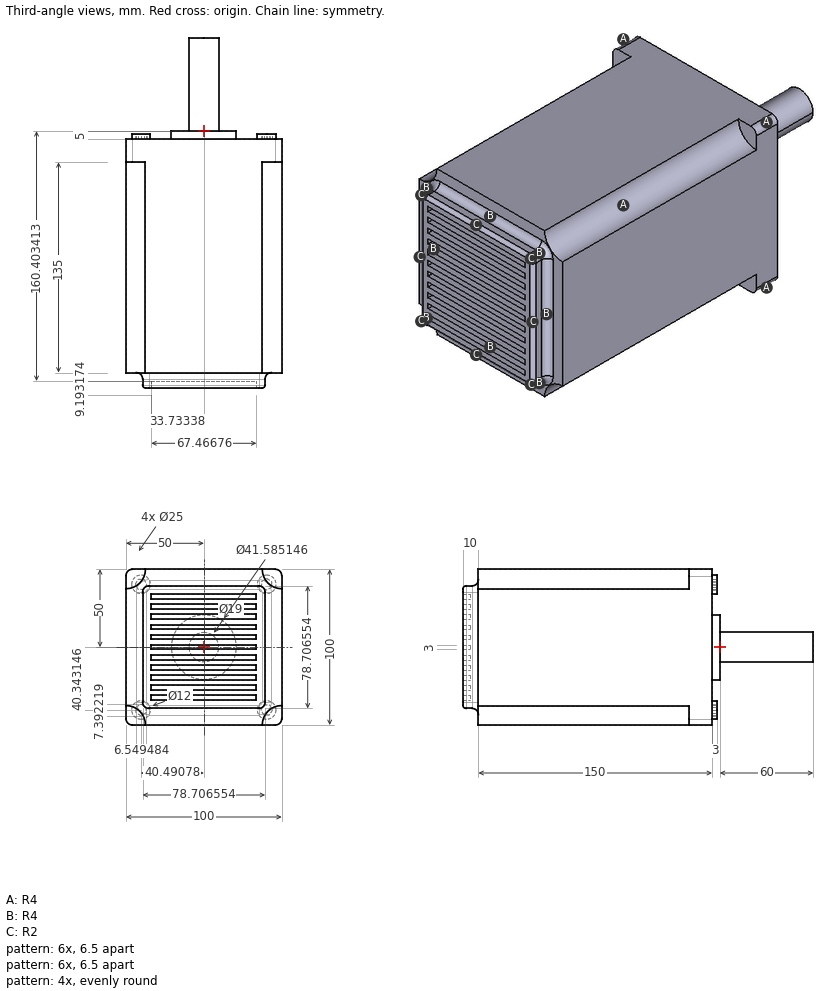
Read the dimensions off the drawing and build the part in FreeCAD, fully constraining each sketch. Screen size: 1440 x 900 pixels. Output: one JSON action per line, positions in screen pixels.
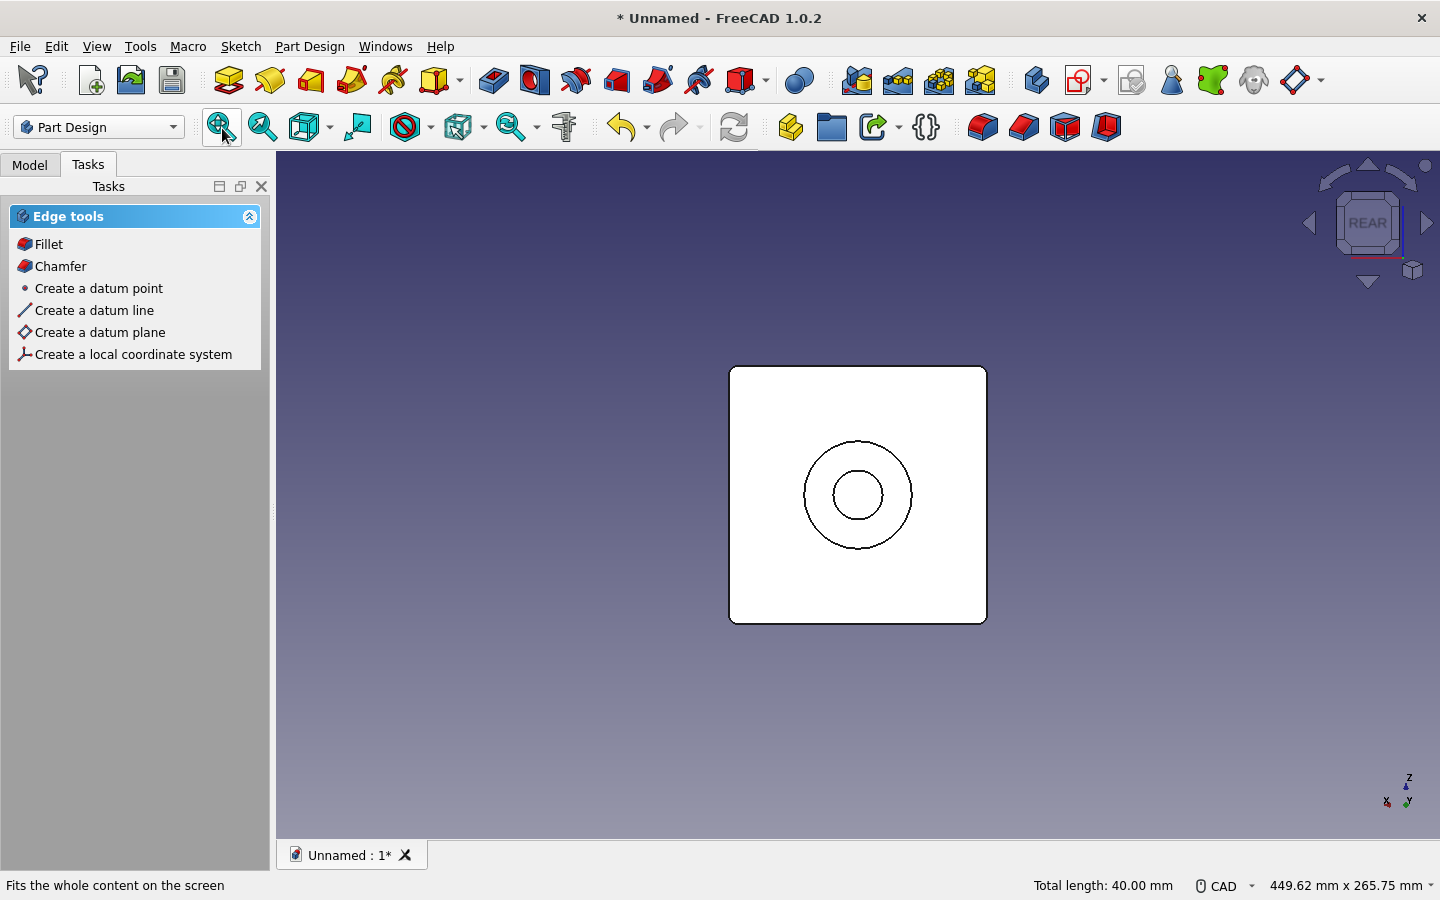
{"action": "key", "text": "6"}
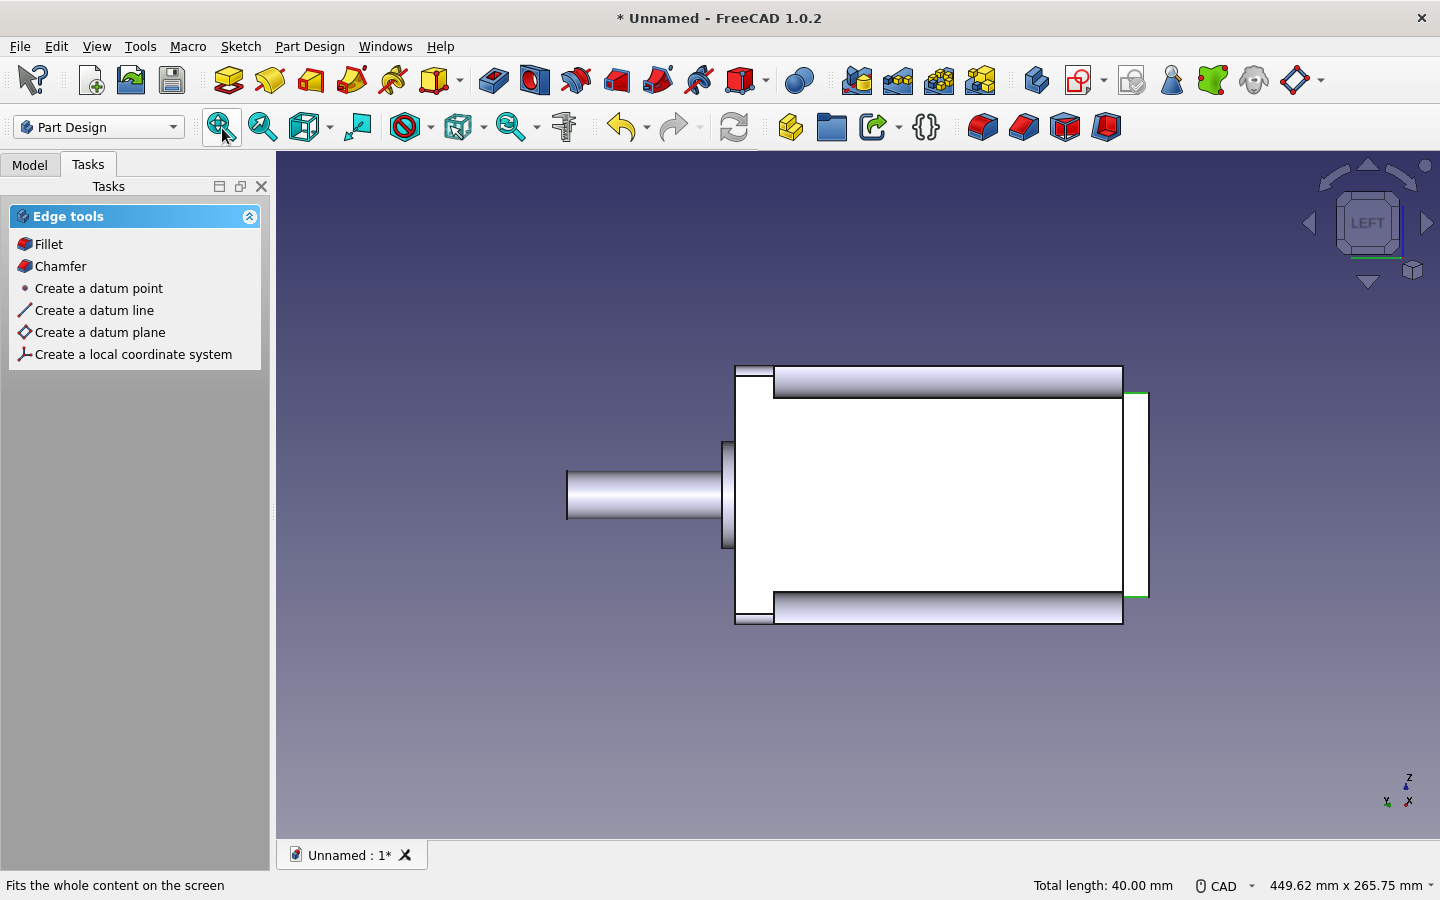
{"action": "key", "text": "v 3"}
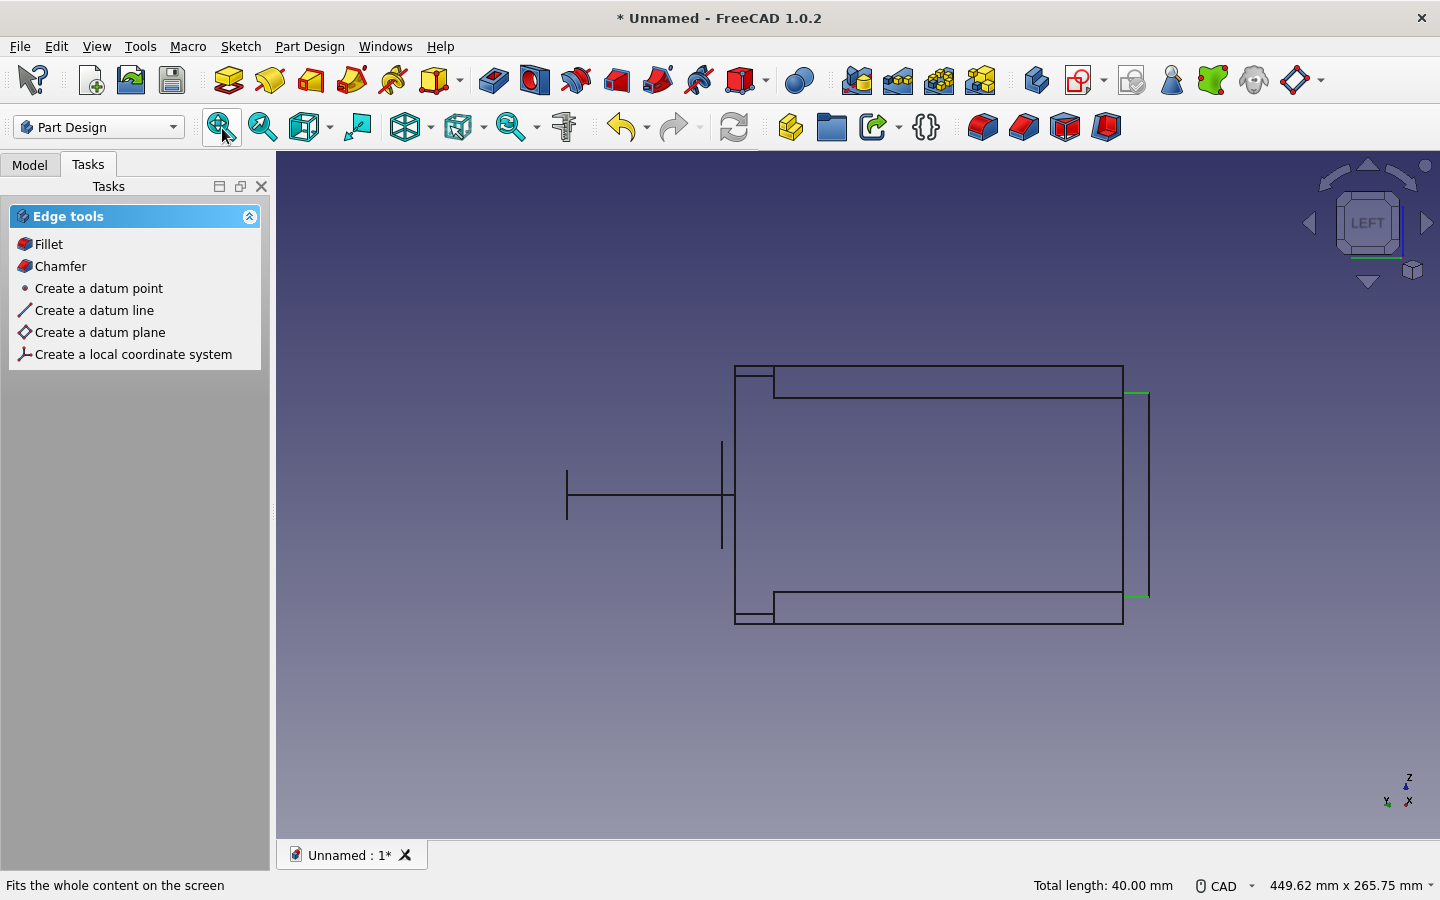
{"action": "key", "text": "0"}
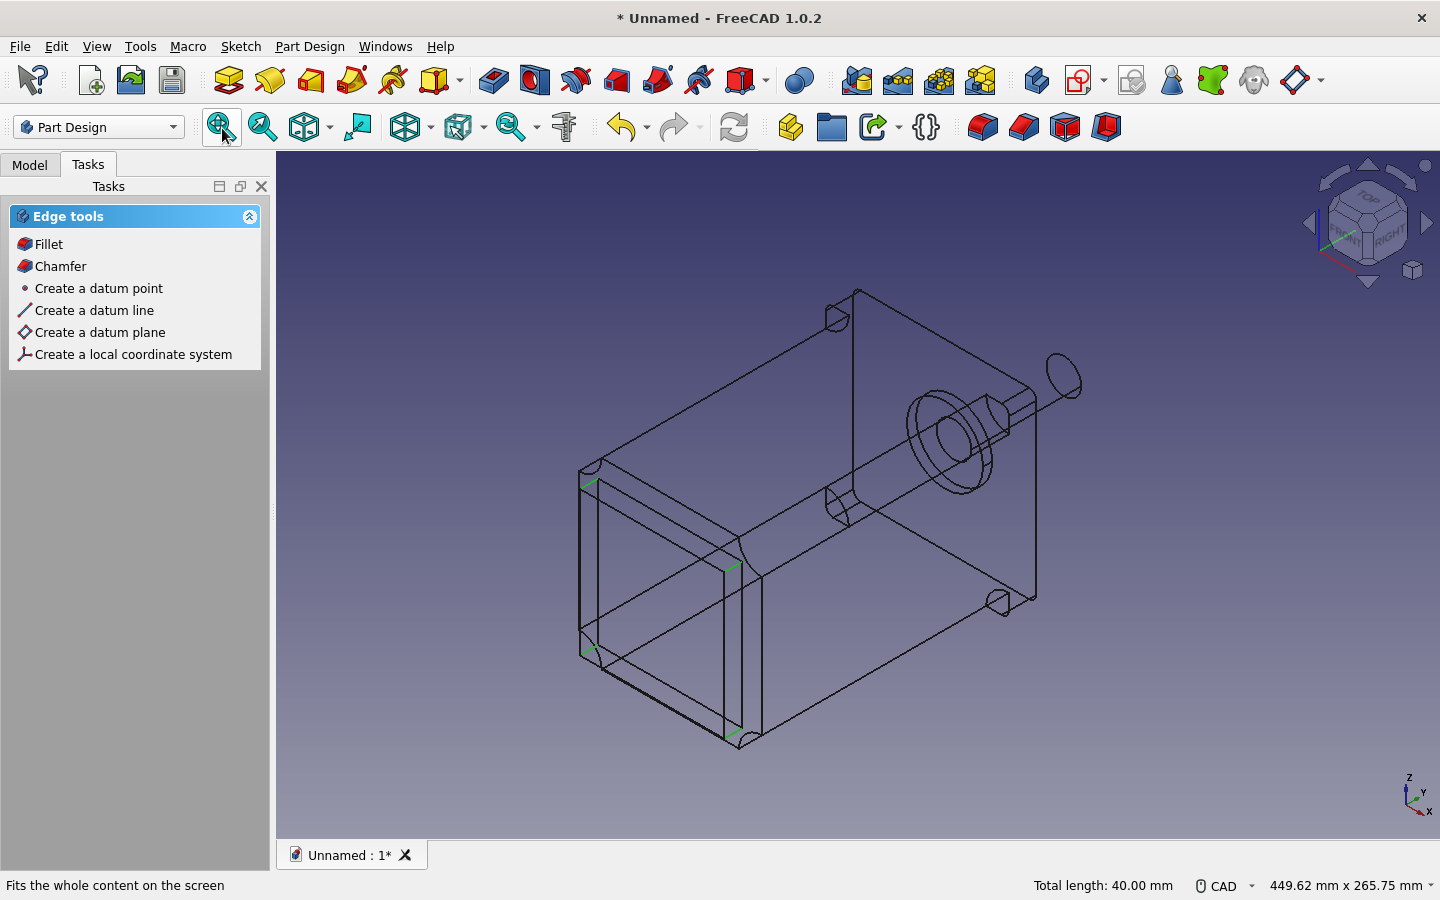
{"action": "left_click", "coordinate": [742, 644], "text": "ctrl"}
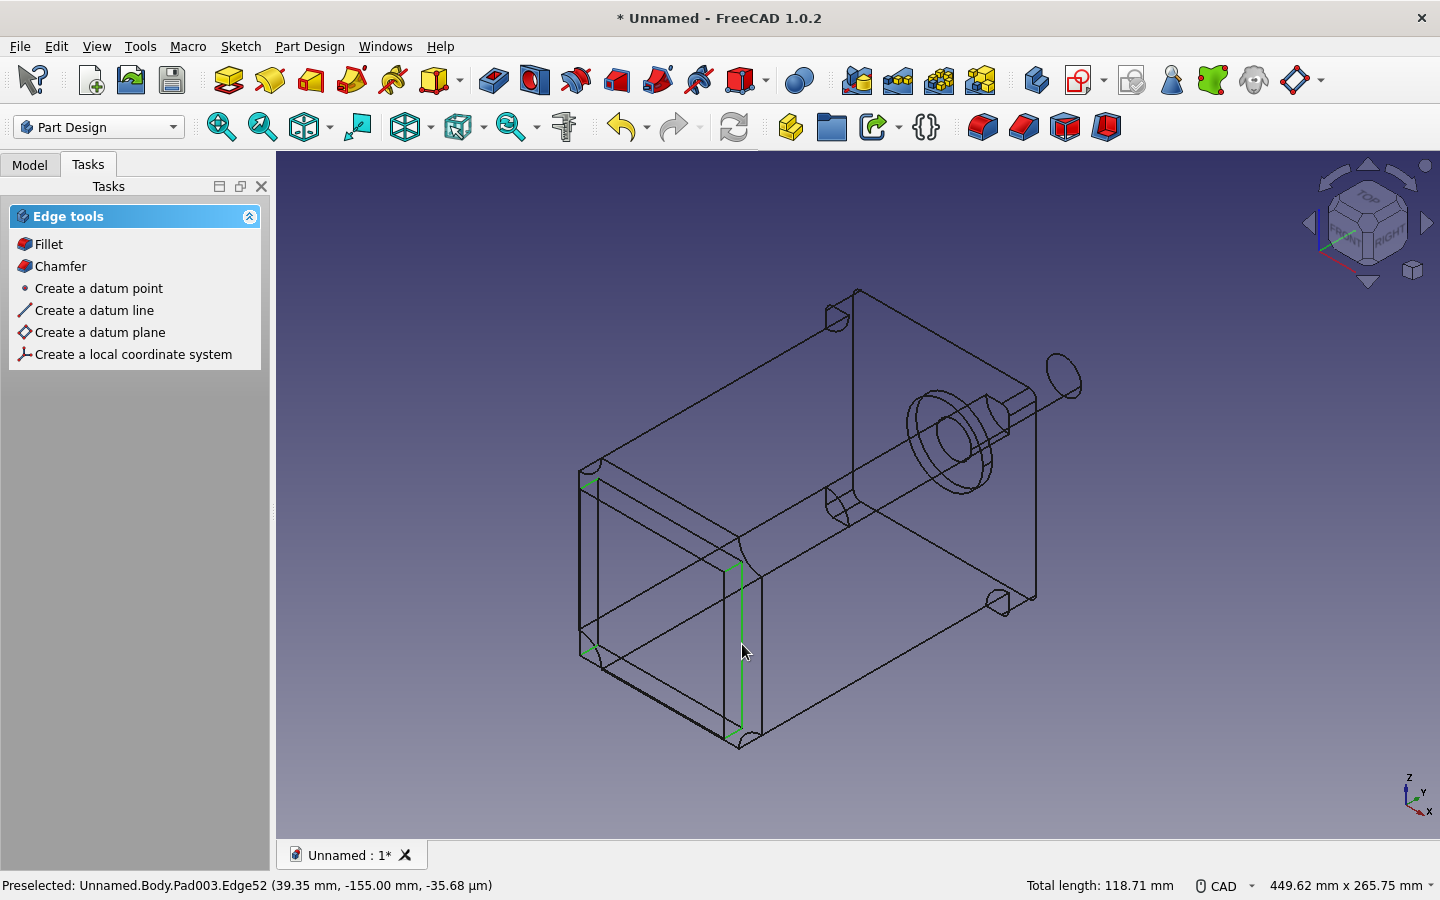
{"action": "left_click", "coordinate": [670, 519], "text": "ctrl"}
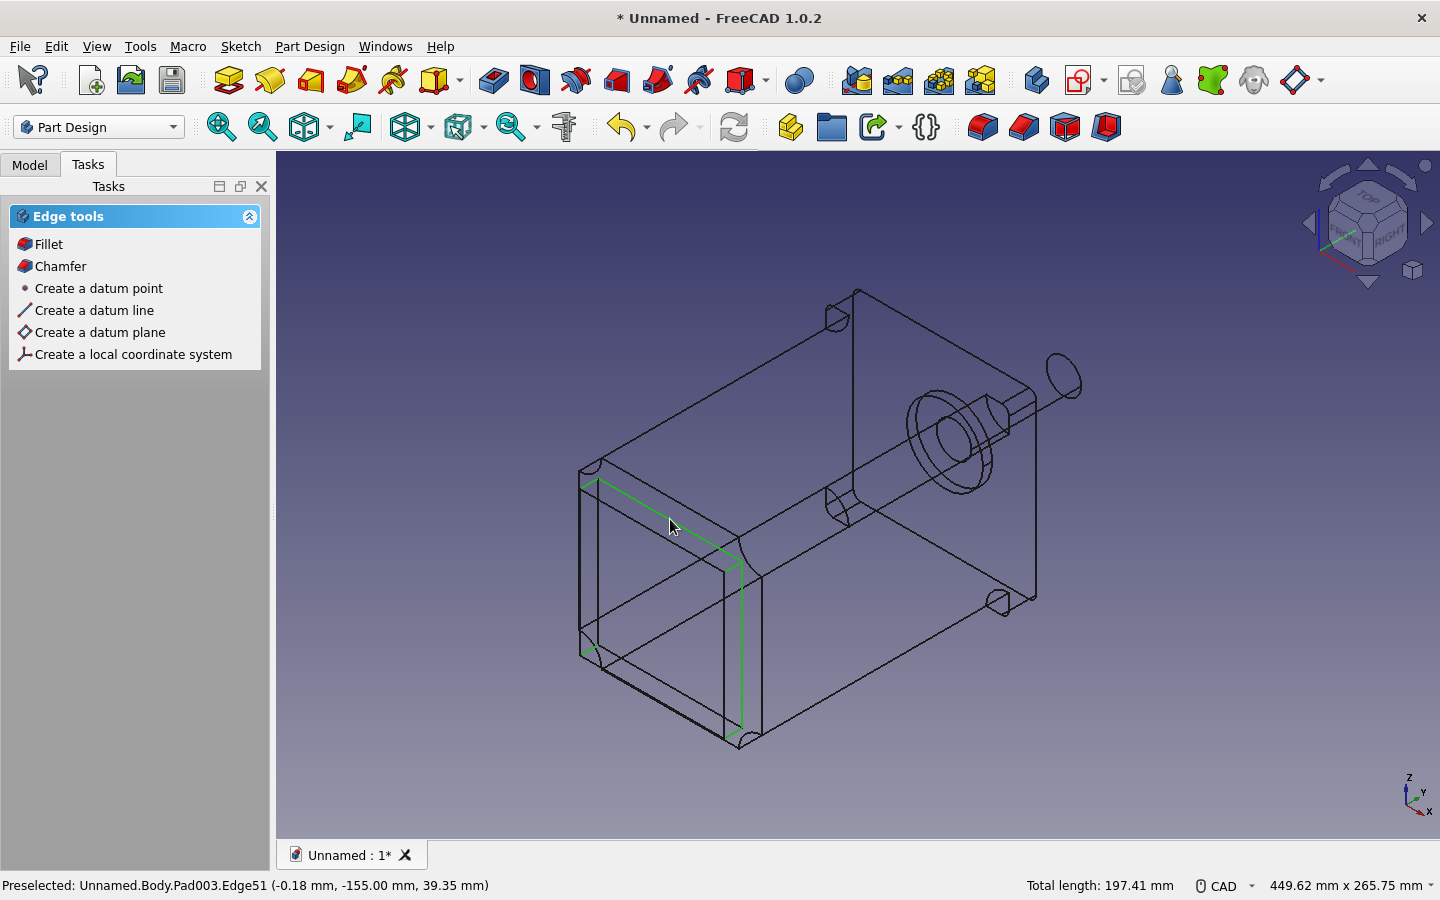
{"action": "left_click", "coordinate": [598, 561], "text": "ctrl"}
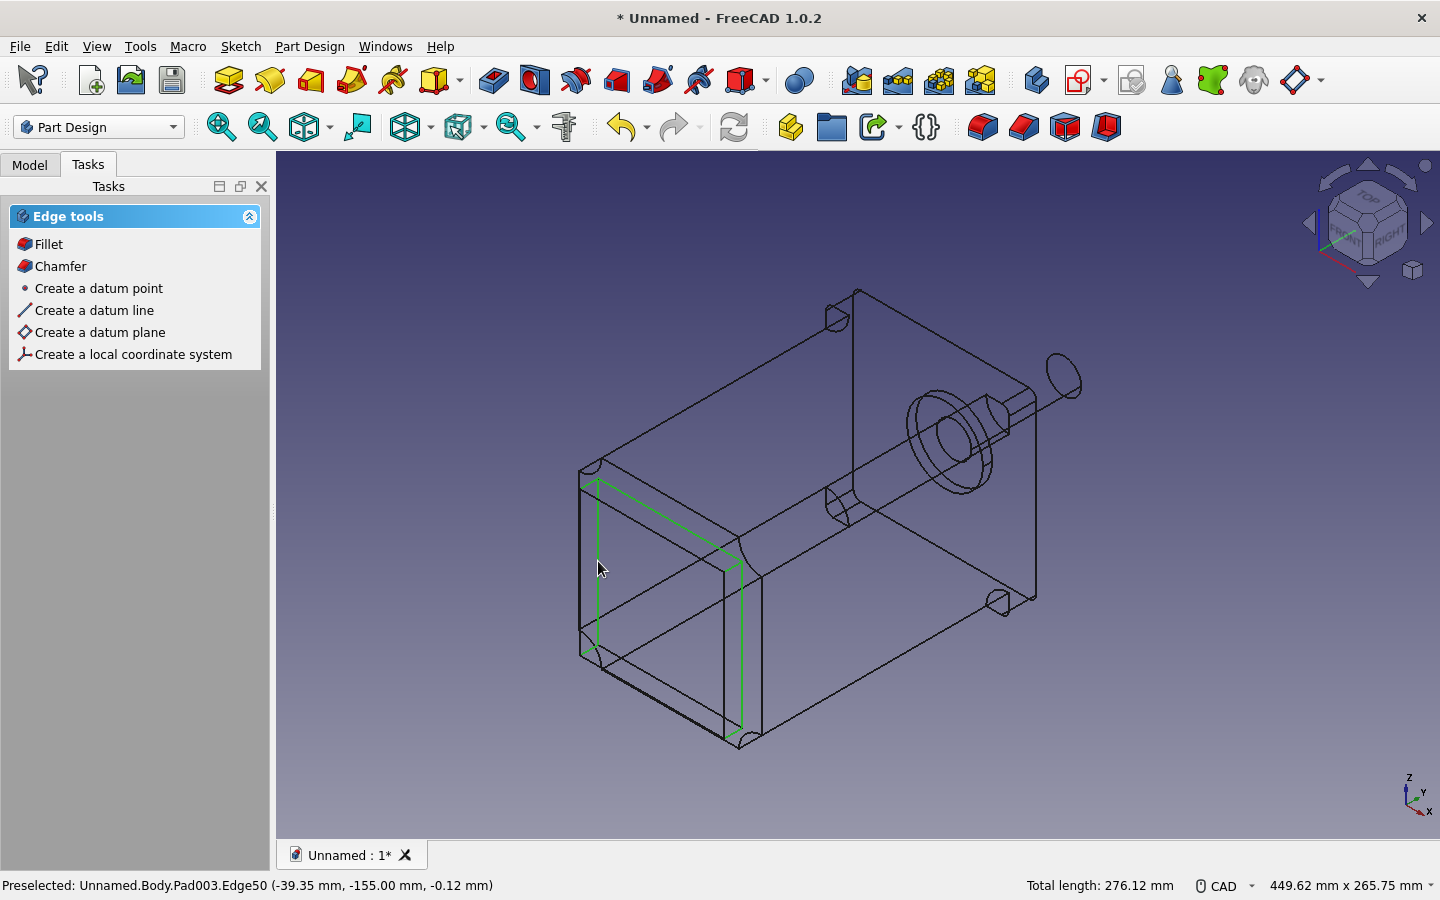
{"action": "left_click", "coordinate": [670, 686], "text": "ctrl"}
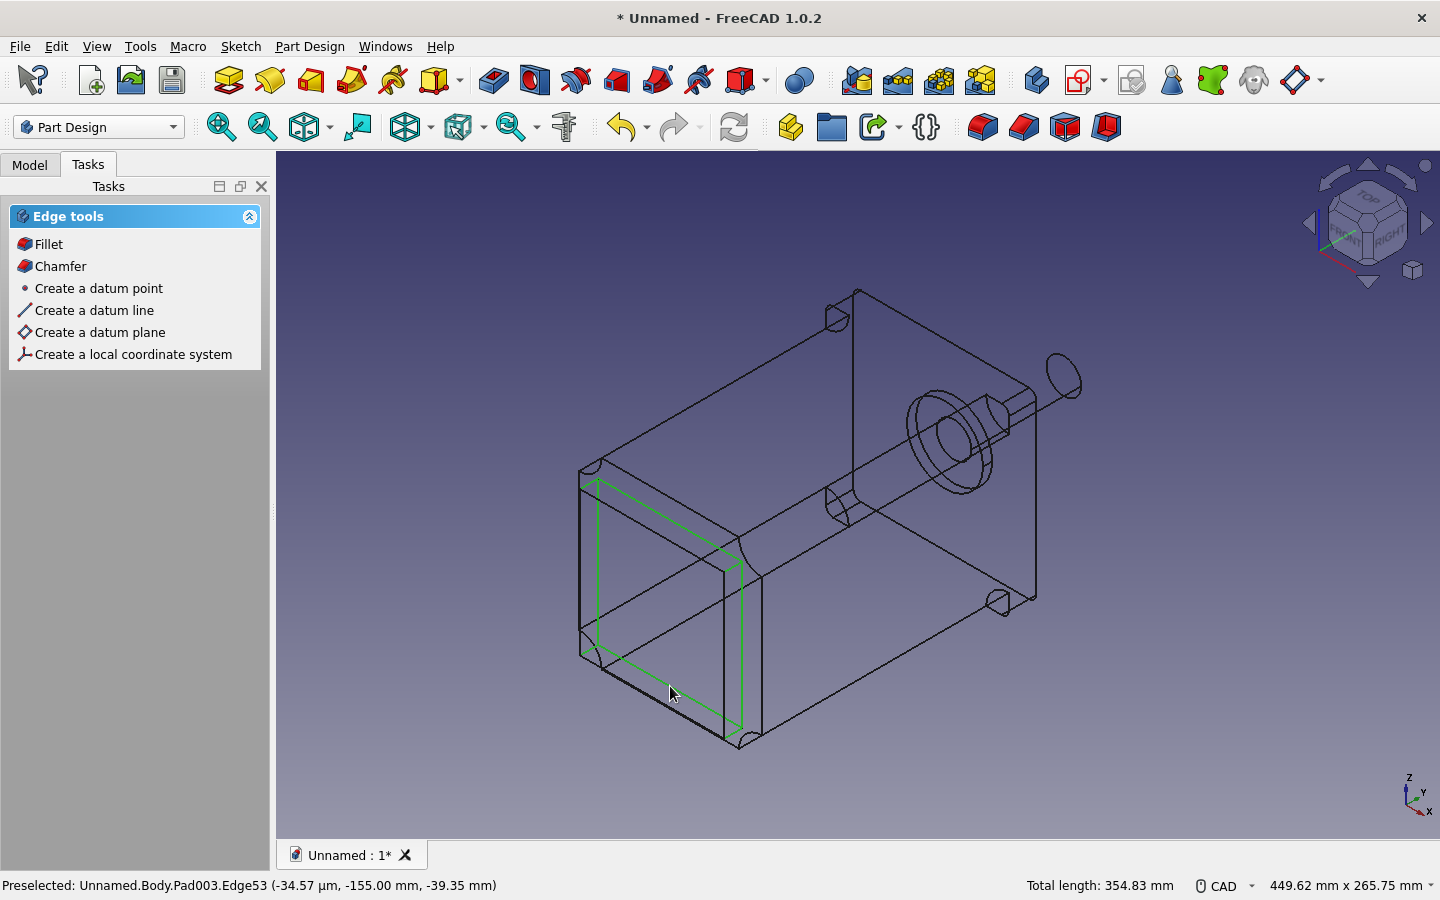
{"action": "key", "text": "v 1"}